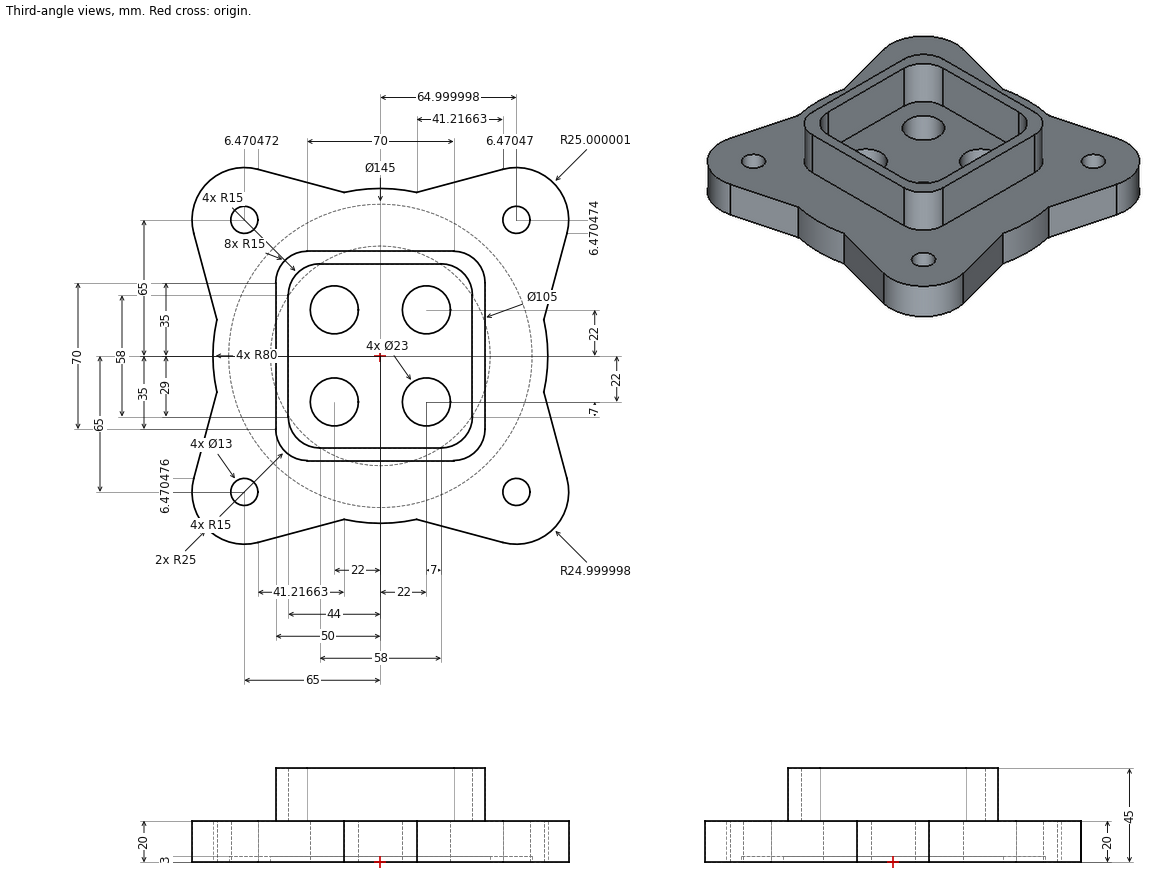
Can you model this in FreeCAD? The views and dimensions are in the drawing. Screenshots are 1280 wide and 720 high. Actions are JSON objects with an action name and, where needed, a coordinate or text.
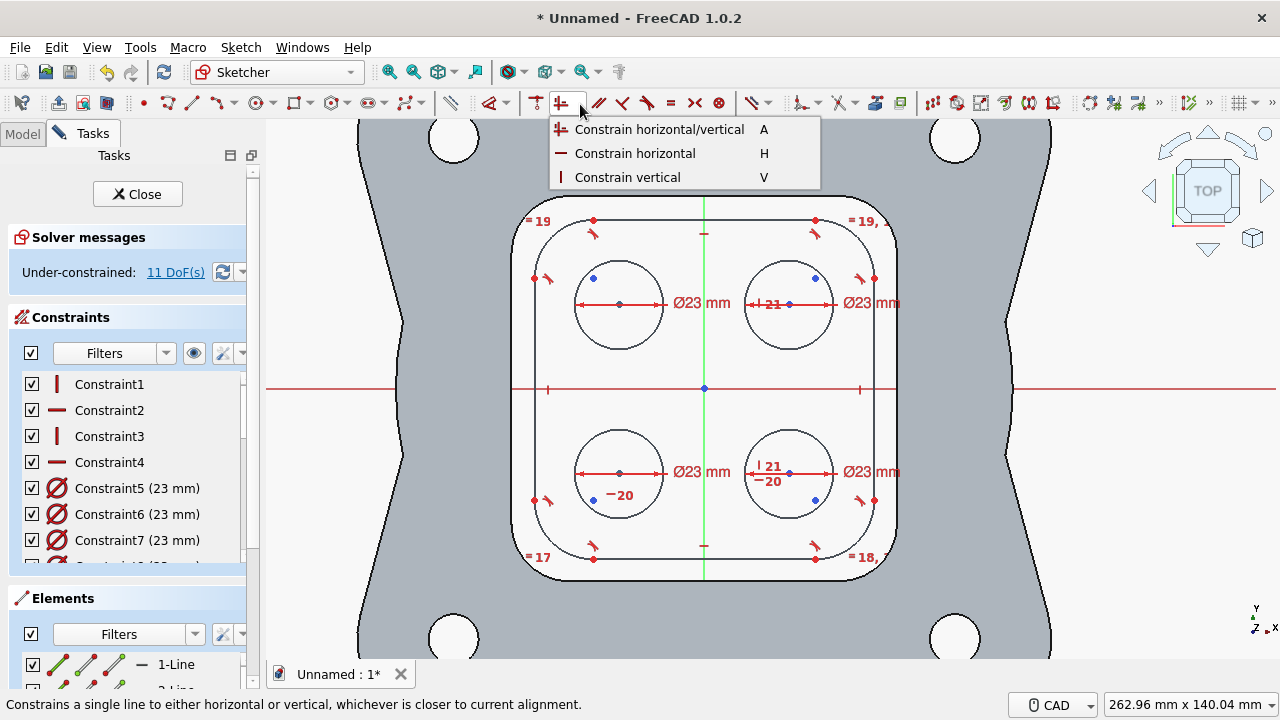
{"action": "left_click", "coordinate": [685, 177]}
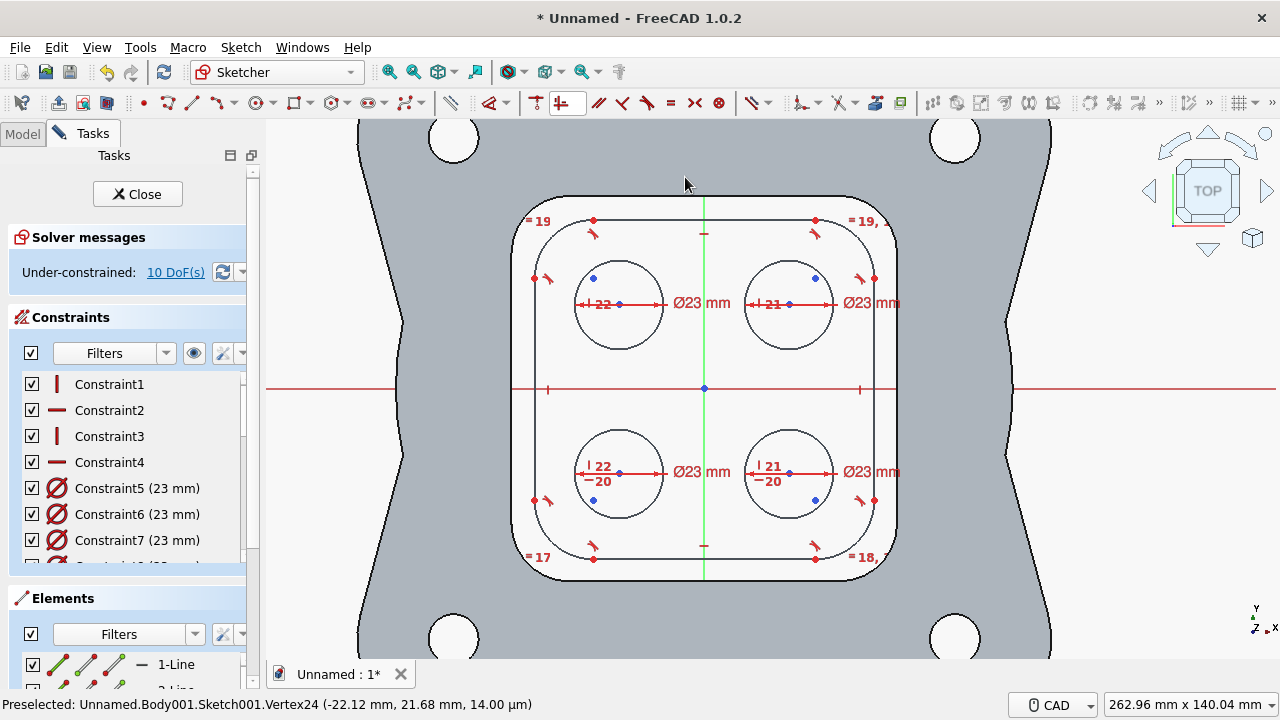
{"action": "left_click", "coordinate": [789, 305]}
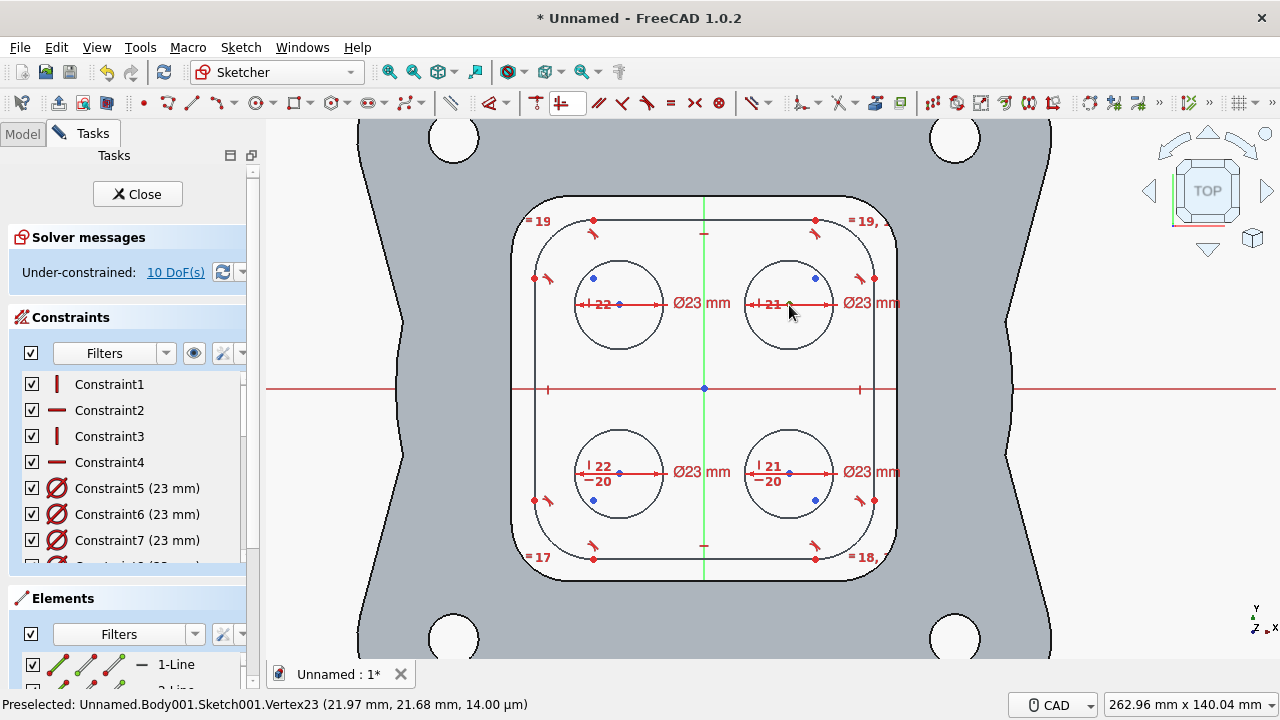
{"action": "left_click", "coordinate": [619, 305]}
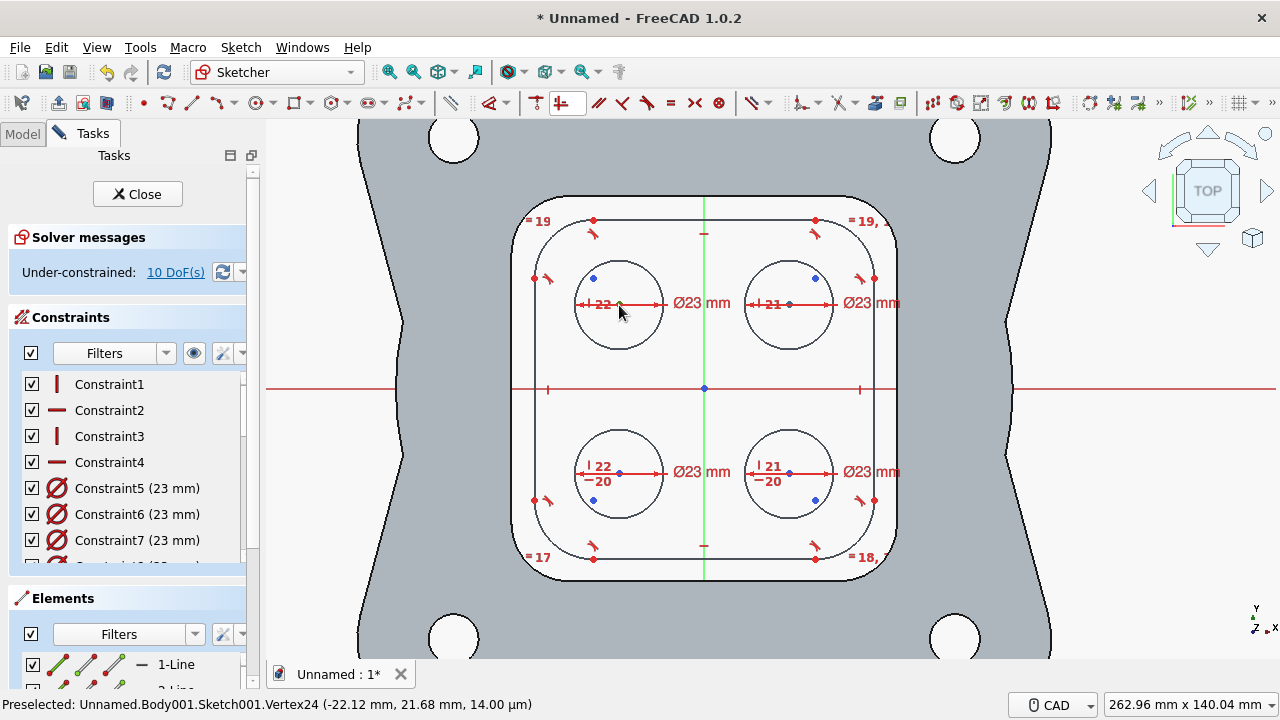
{"action": "left_click", "coordinate": [580, 104]}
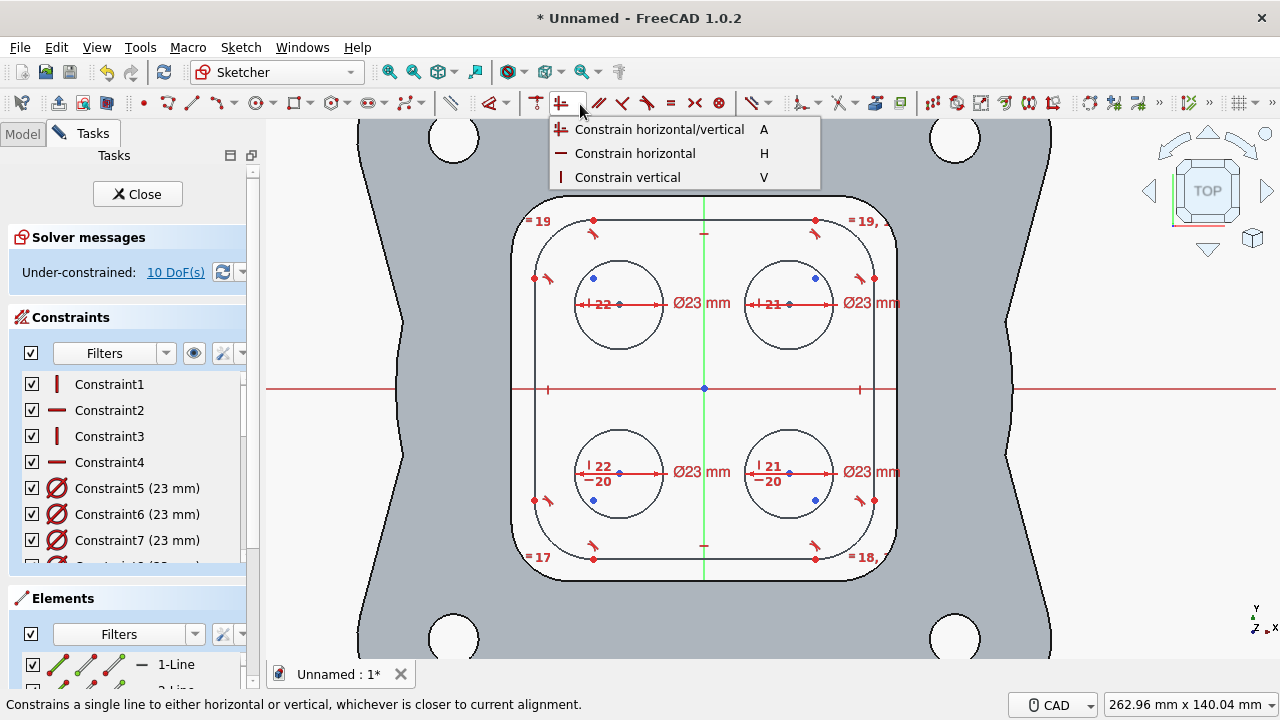
{"action": "left_click", "coordinate": [685, 153]}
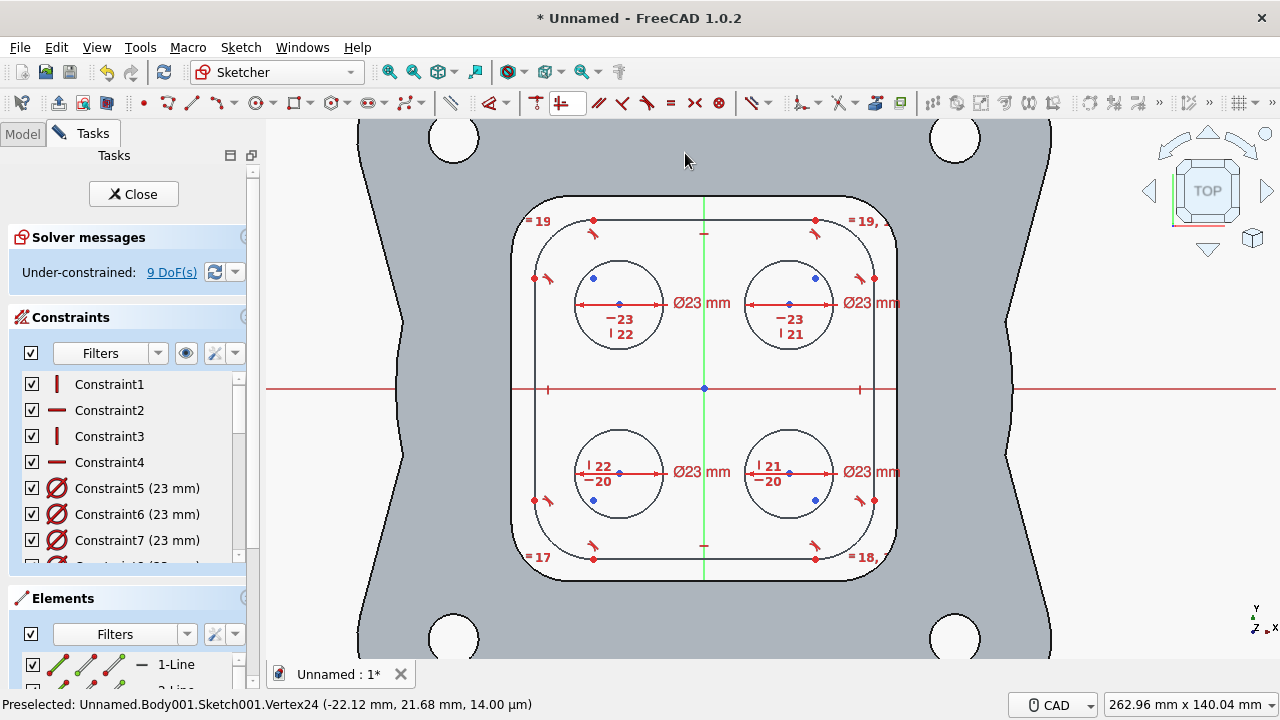
{"action": "key", "text": "d"}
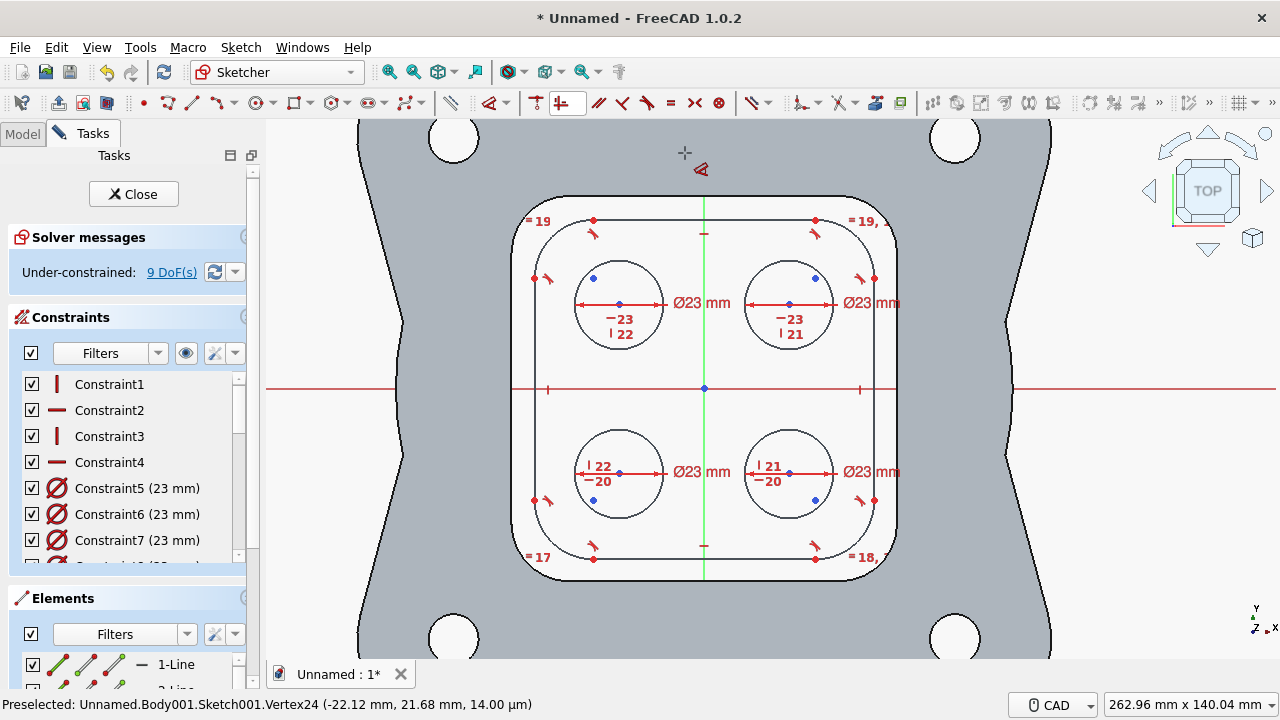
{"action": "left_click", "coordinate": [541, 527]}
{"action": "left_click", "coordinate": [512, 541]}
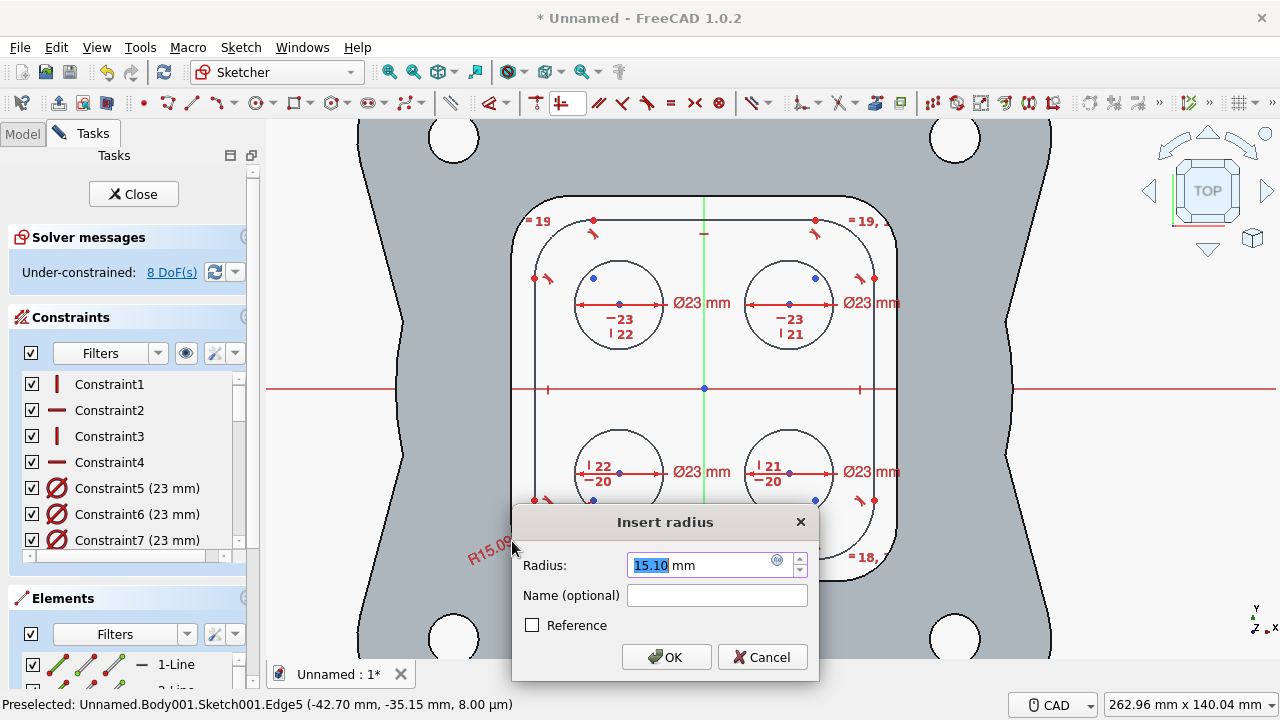
{"action": "type", "text": "15"}
{"action": "key", "text": "Return"}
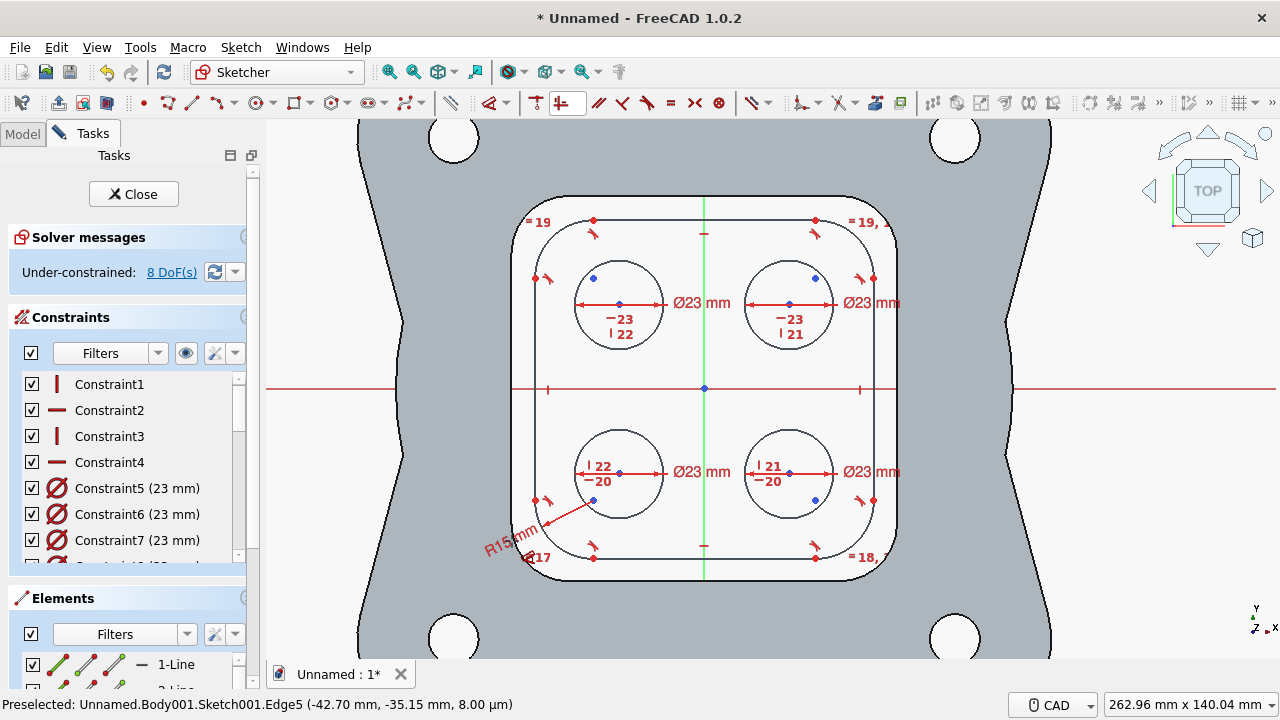
{"action": "left_click", "coordinate": [535, 345]}
{"action": "left_click", "coordinate": [501, 338]}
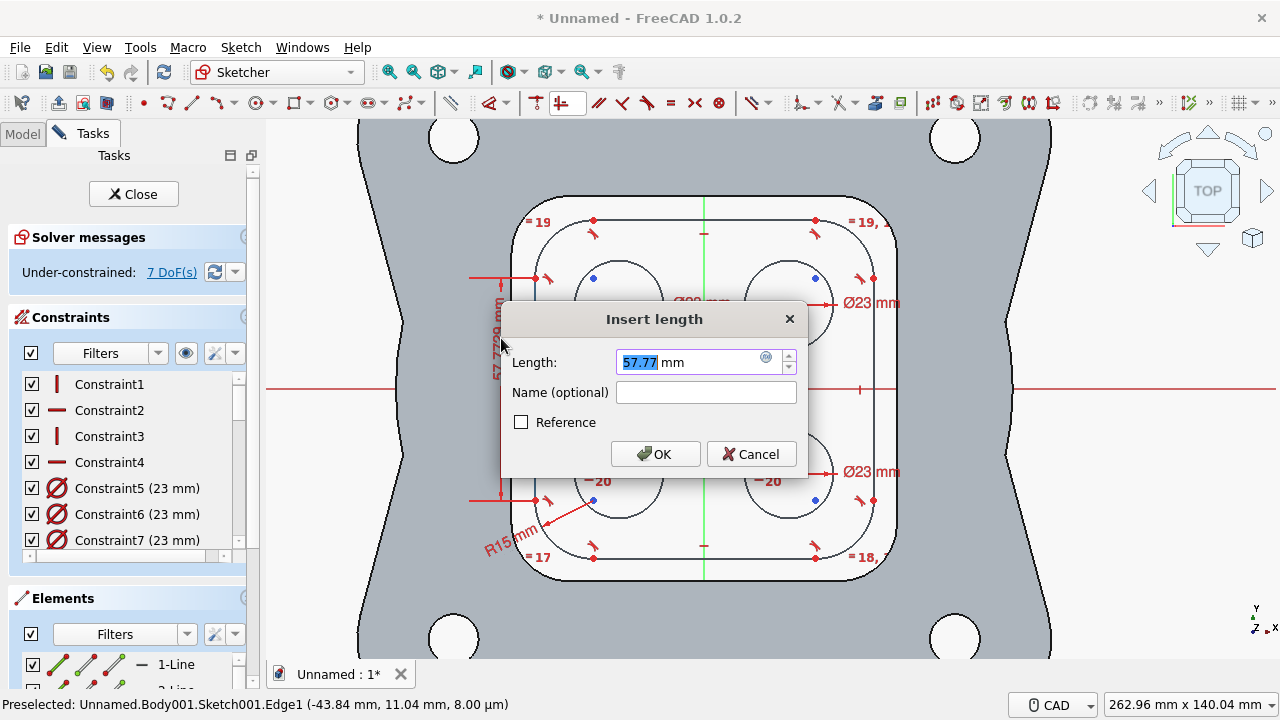
{"action": "type", "text": "58"}
{"action": "key", "text": "Return"}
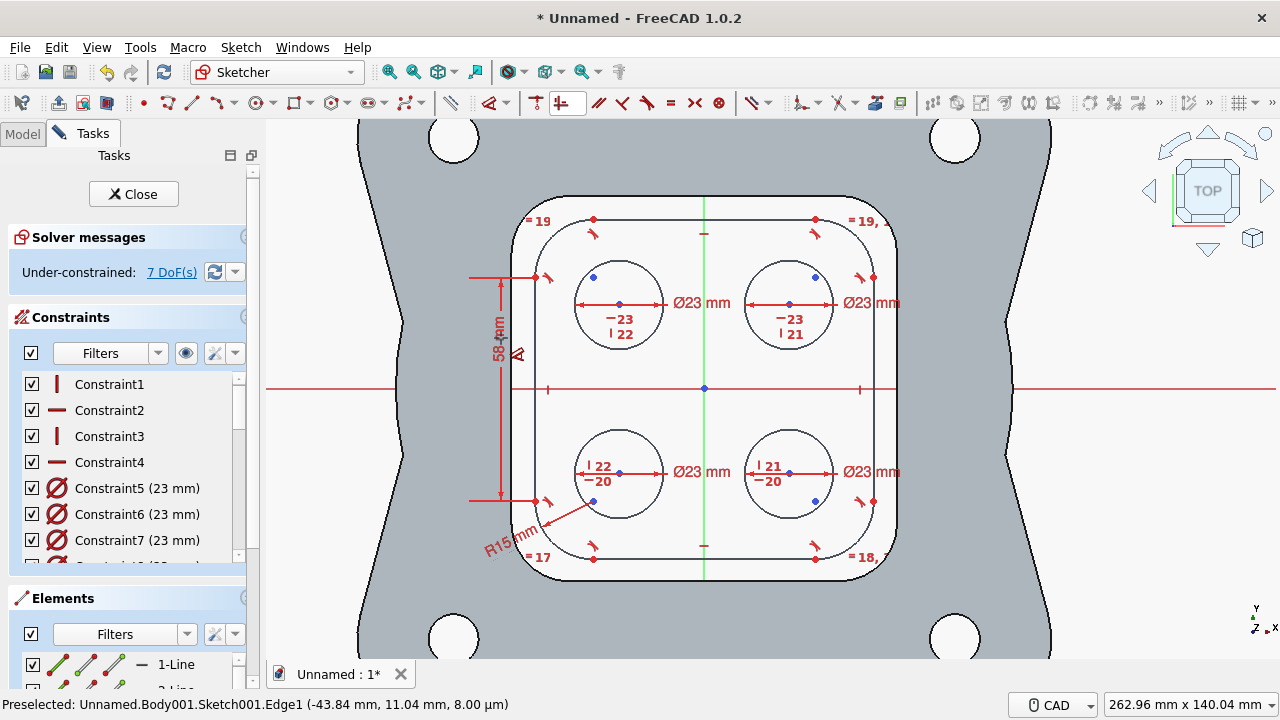
{"action": "left_click", "coordinate": [660, 559]}
{"action": "left_click", "coordinate": [653, 593]}